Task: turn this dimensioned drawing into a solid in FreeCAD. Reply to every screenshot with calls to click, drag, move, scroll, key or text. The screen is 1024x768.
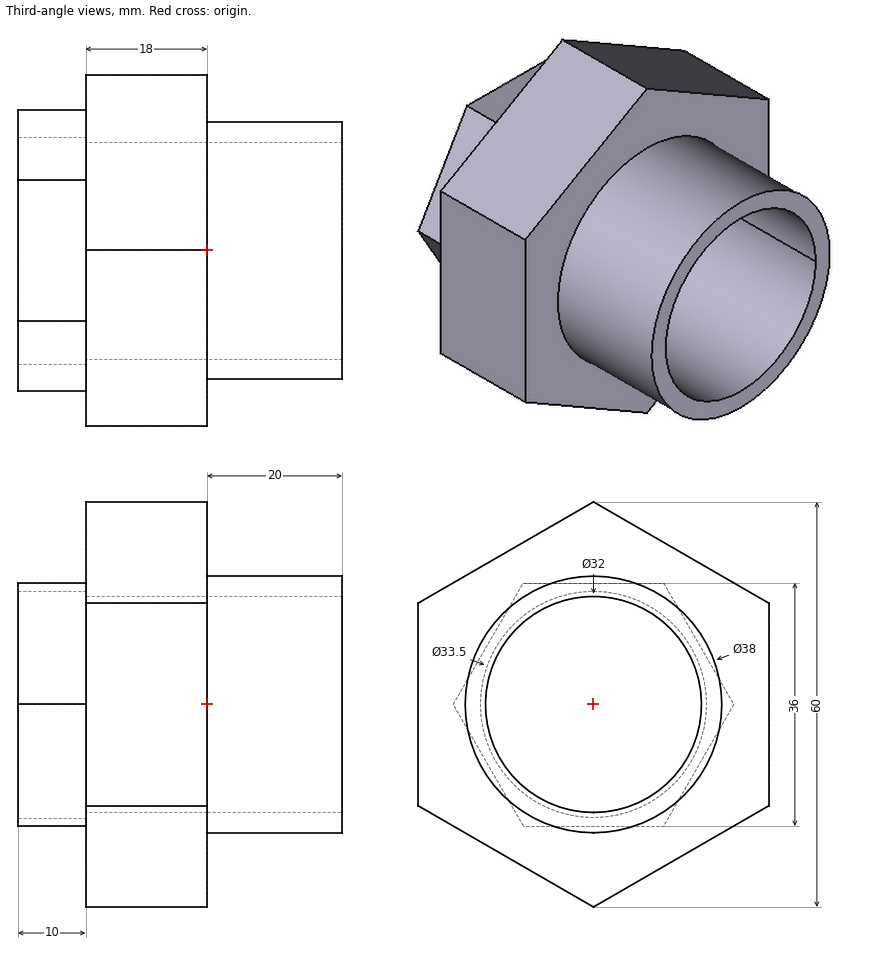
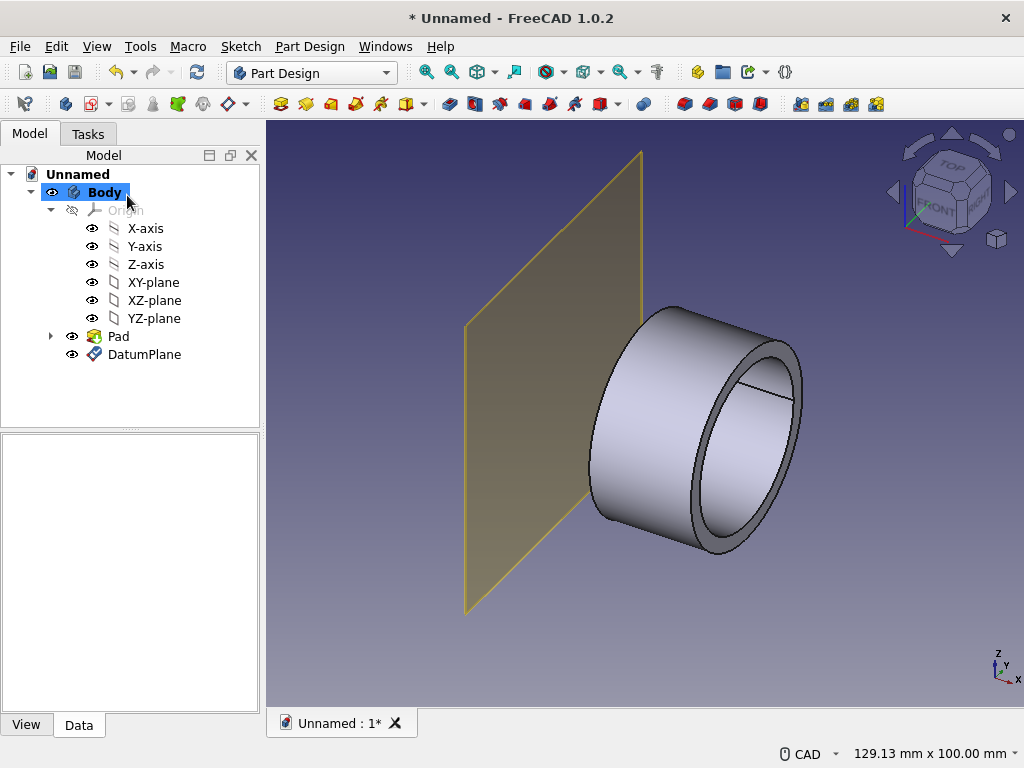
click(117, 354)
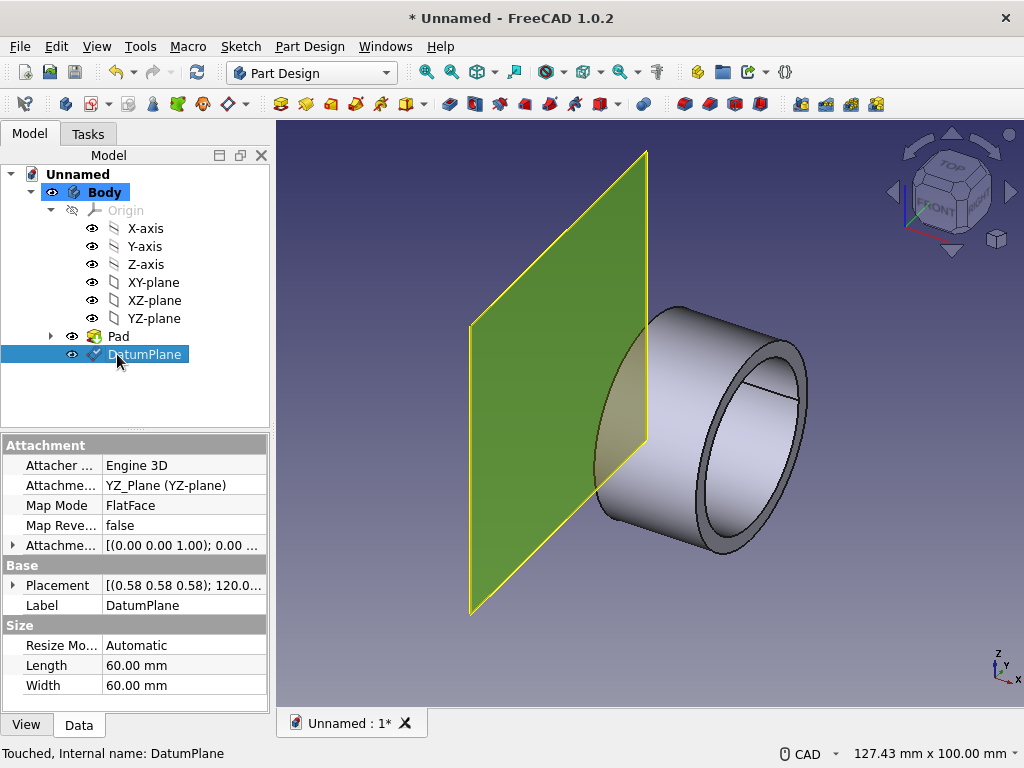
click(90, 104)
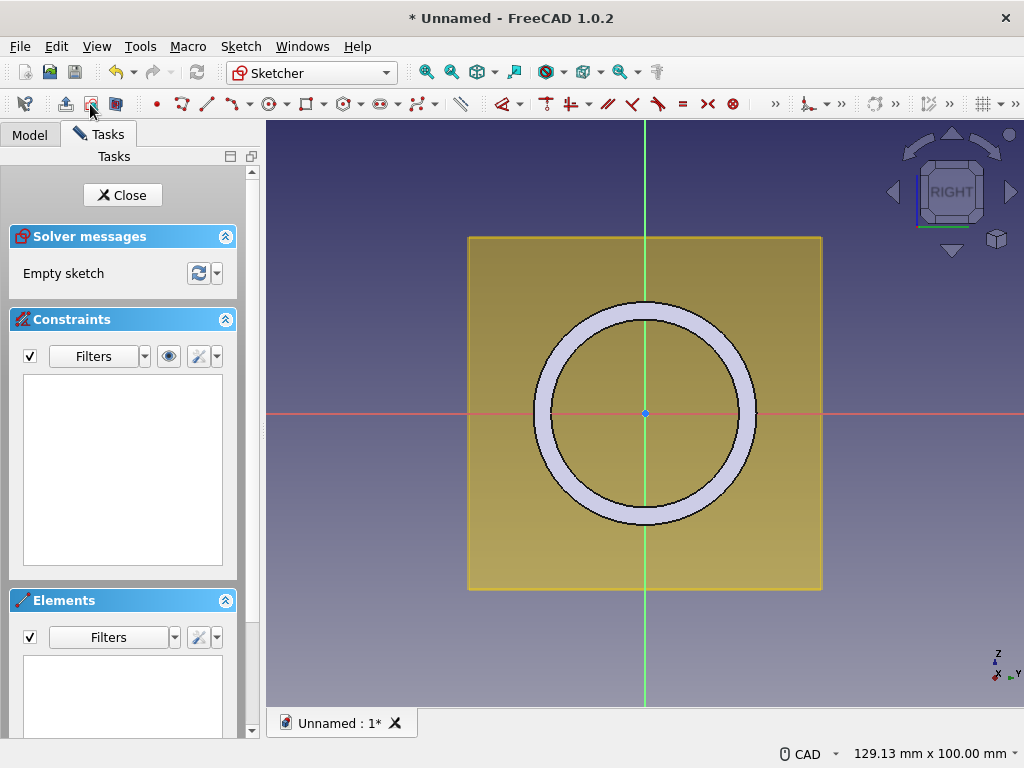
key(q)
key(s)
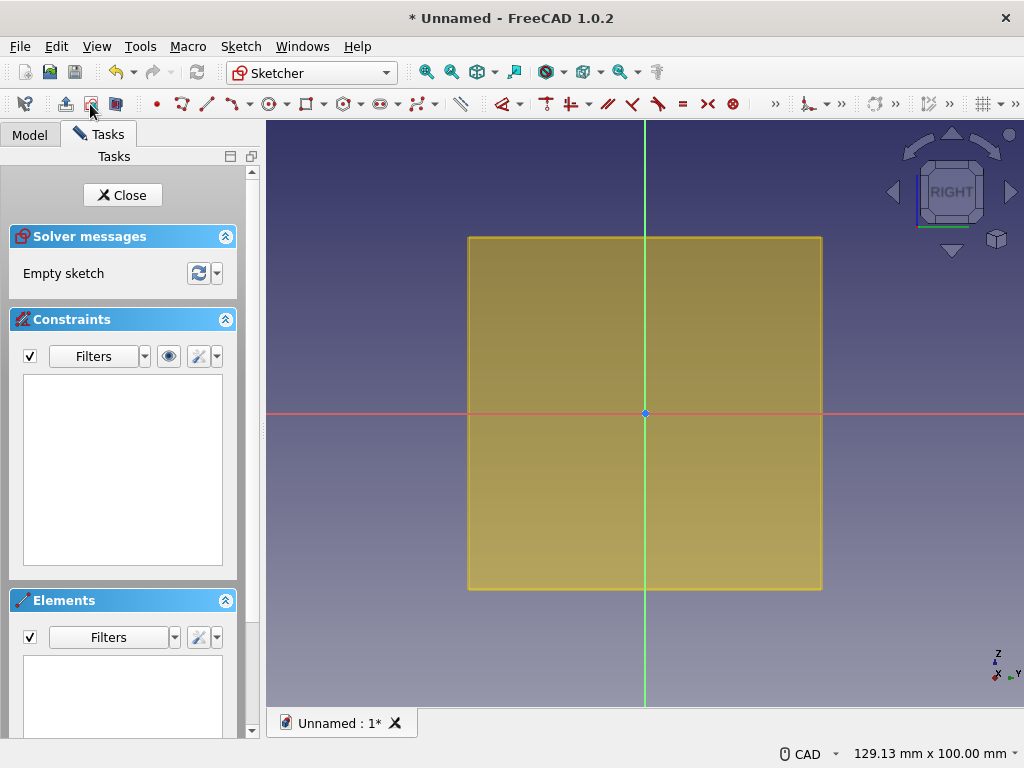
key(g)
key(p)
key(6)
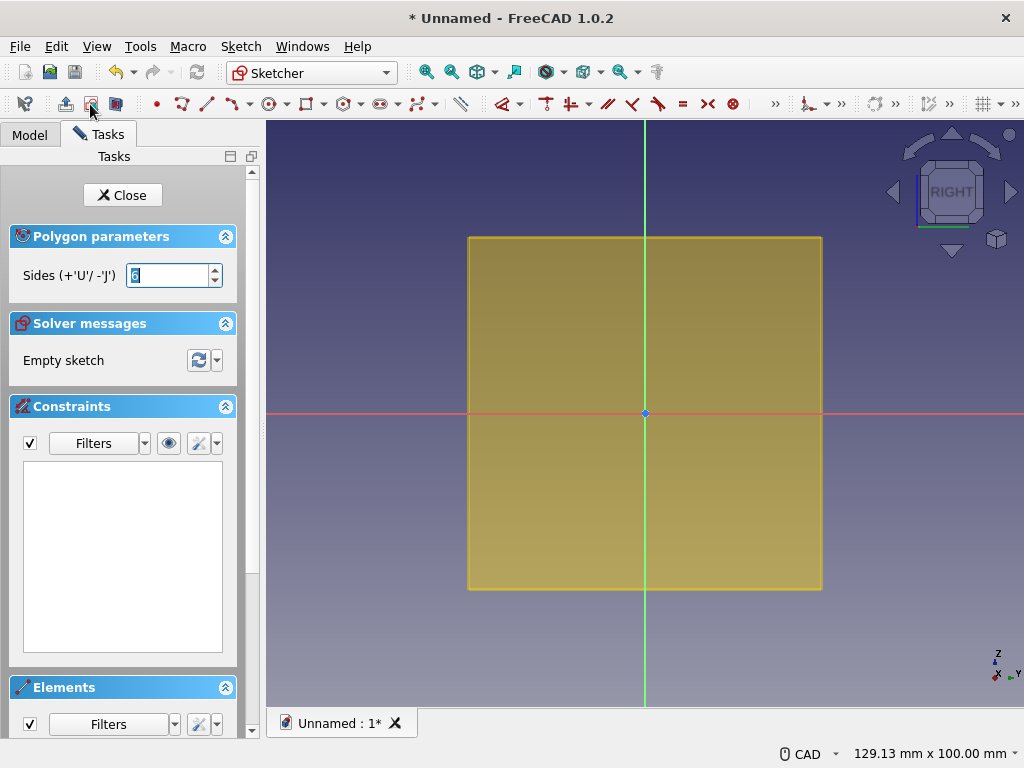
click(645, 414)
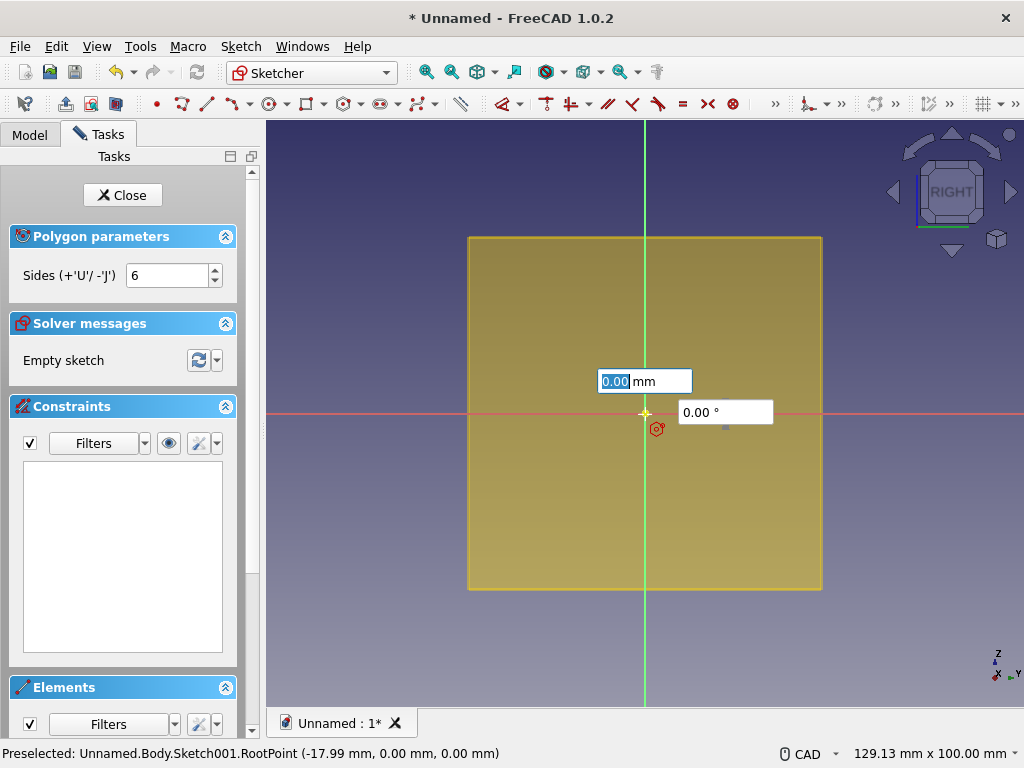
click(645, 237)
right_click(645, 237)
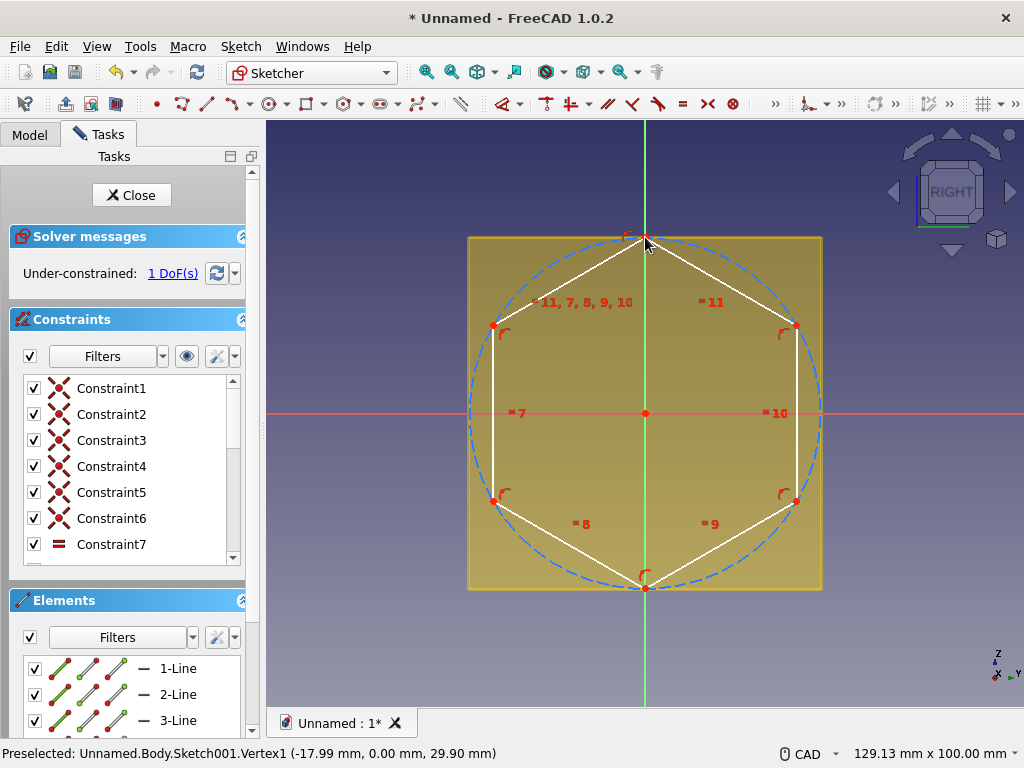
key(g)
key(c)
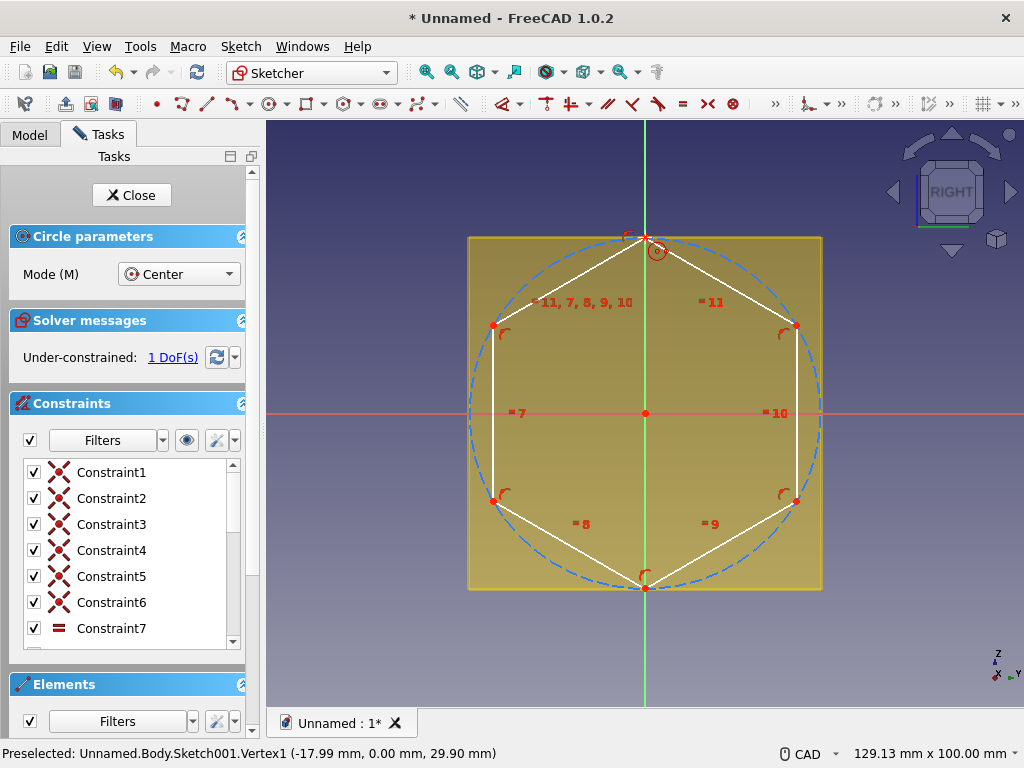
click(645, 414)
click(711, 347)
key(Escape)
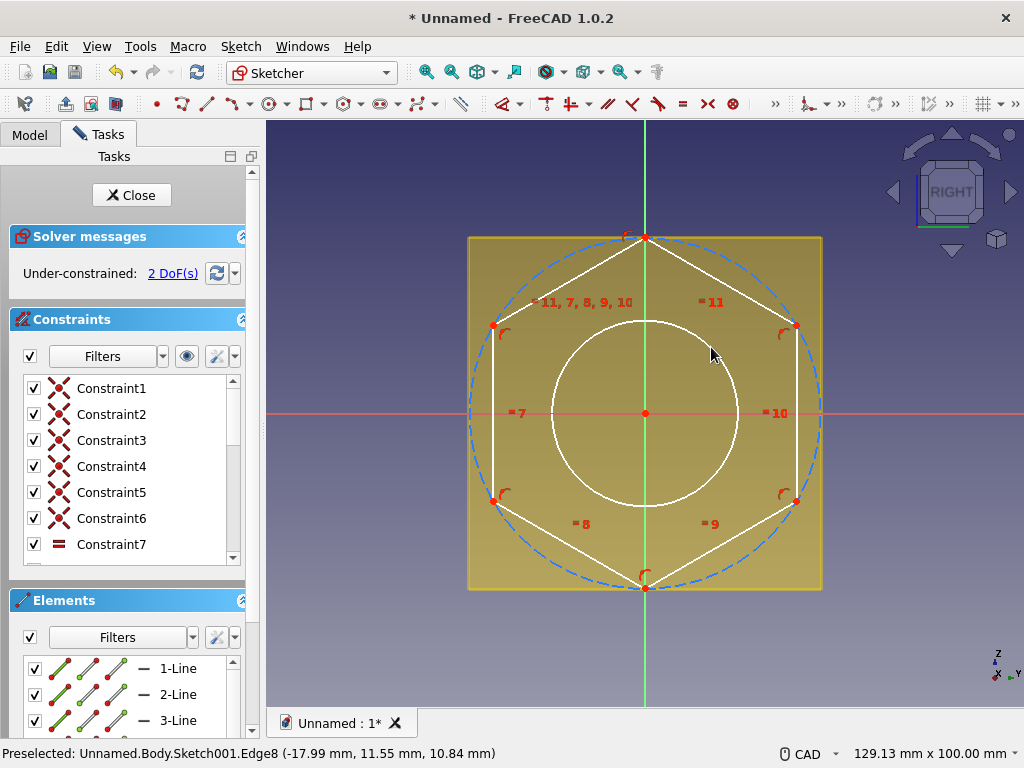
click(711, 348)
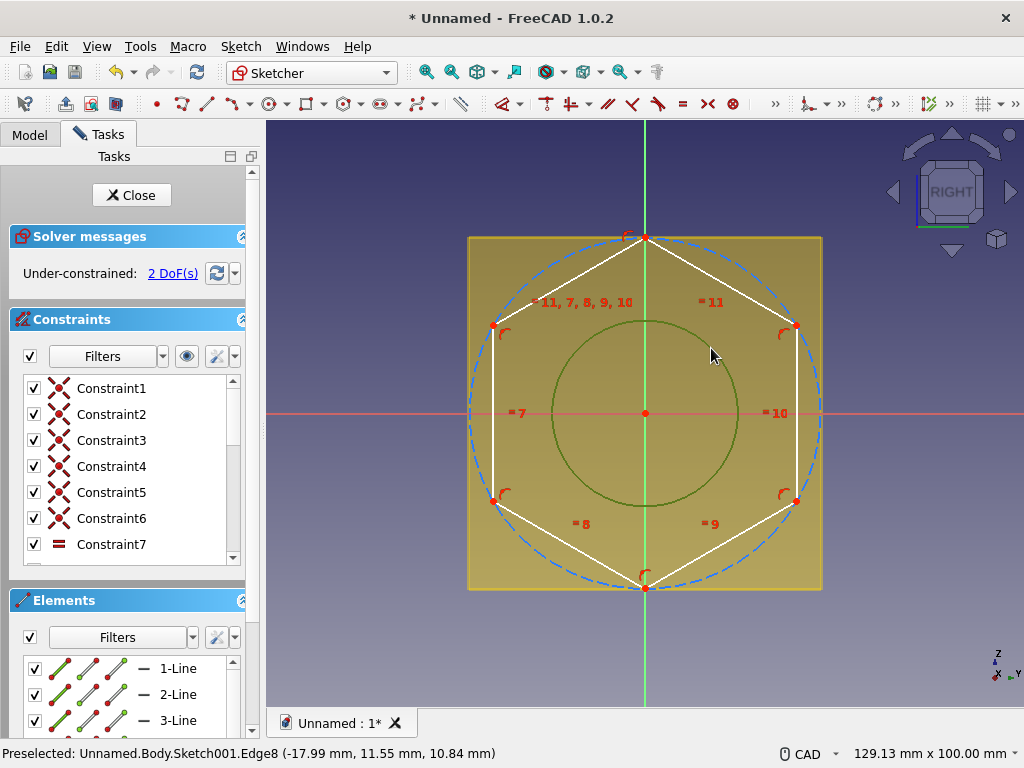
key(k)
key(o)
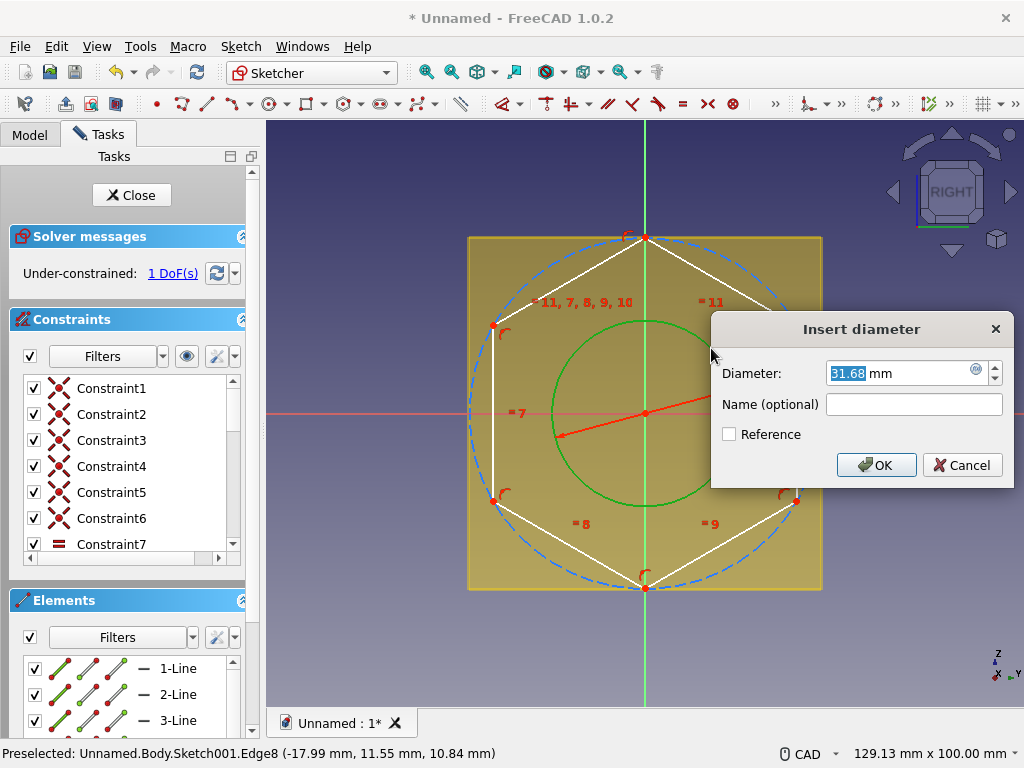
text(32)
key(Return)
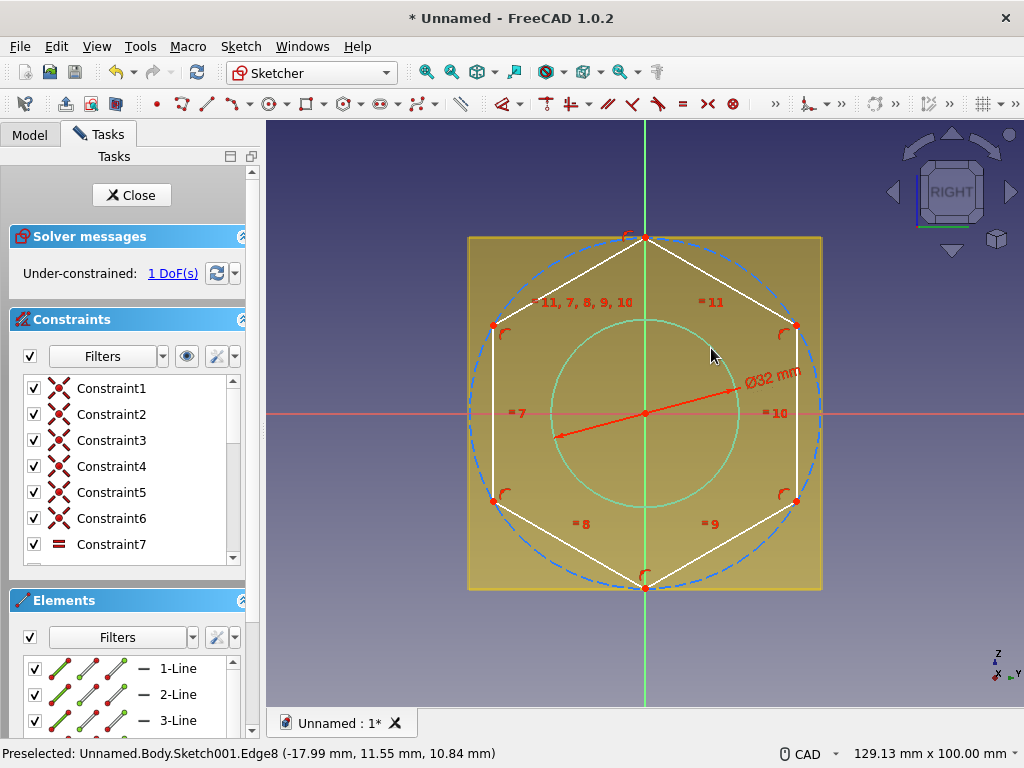
click(645, 589)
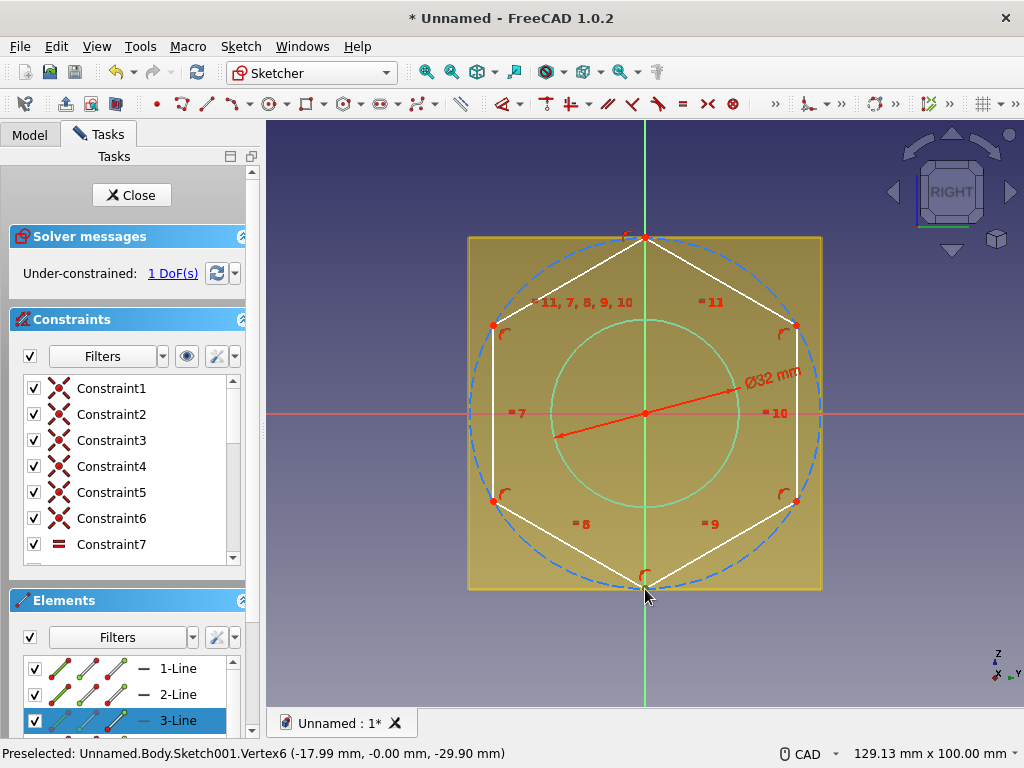
click(645, 238)